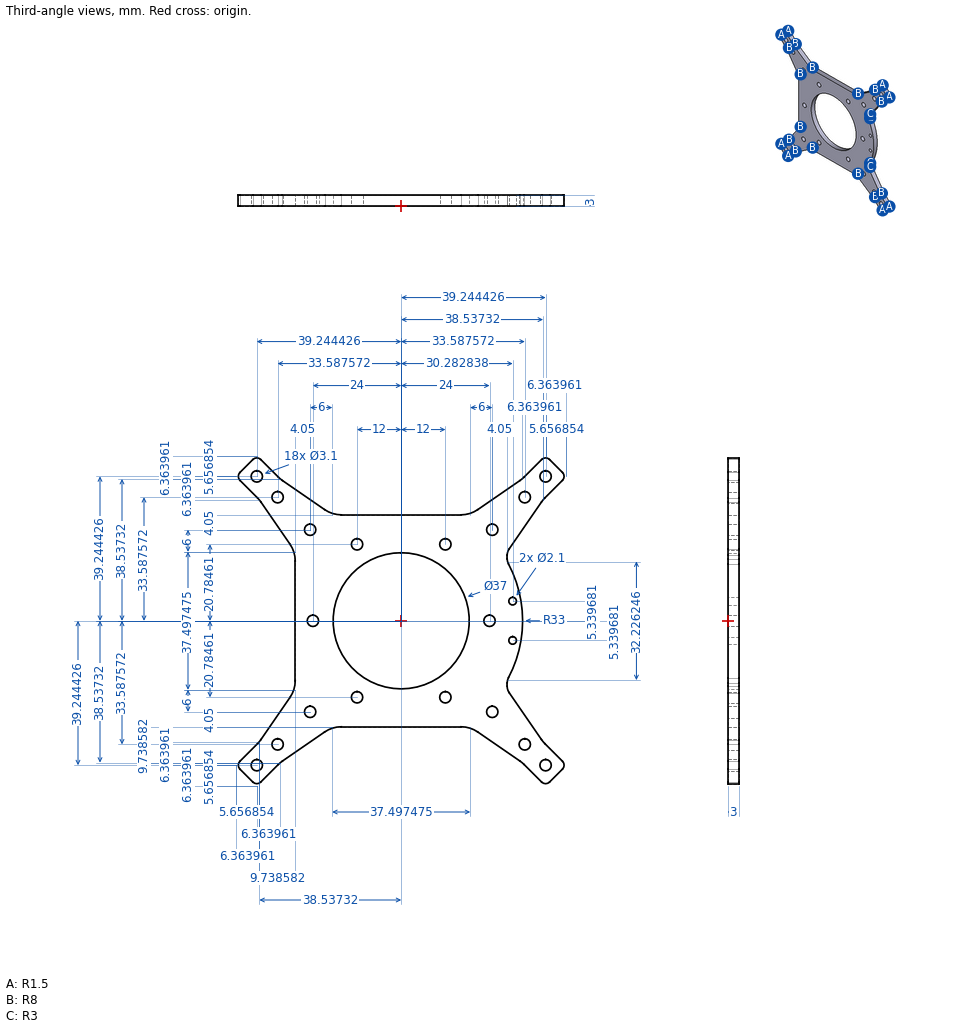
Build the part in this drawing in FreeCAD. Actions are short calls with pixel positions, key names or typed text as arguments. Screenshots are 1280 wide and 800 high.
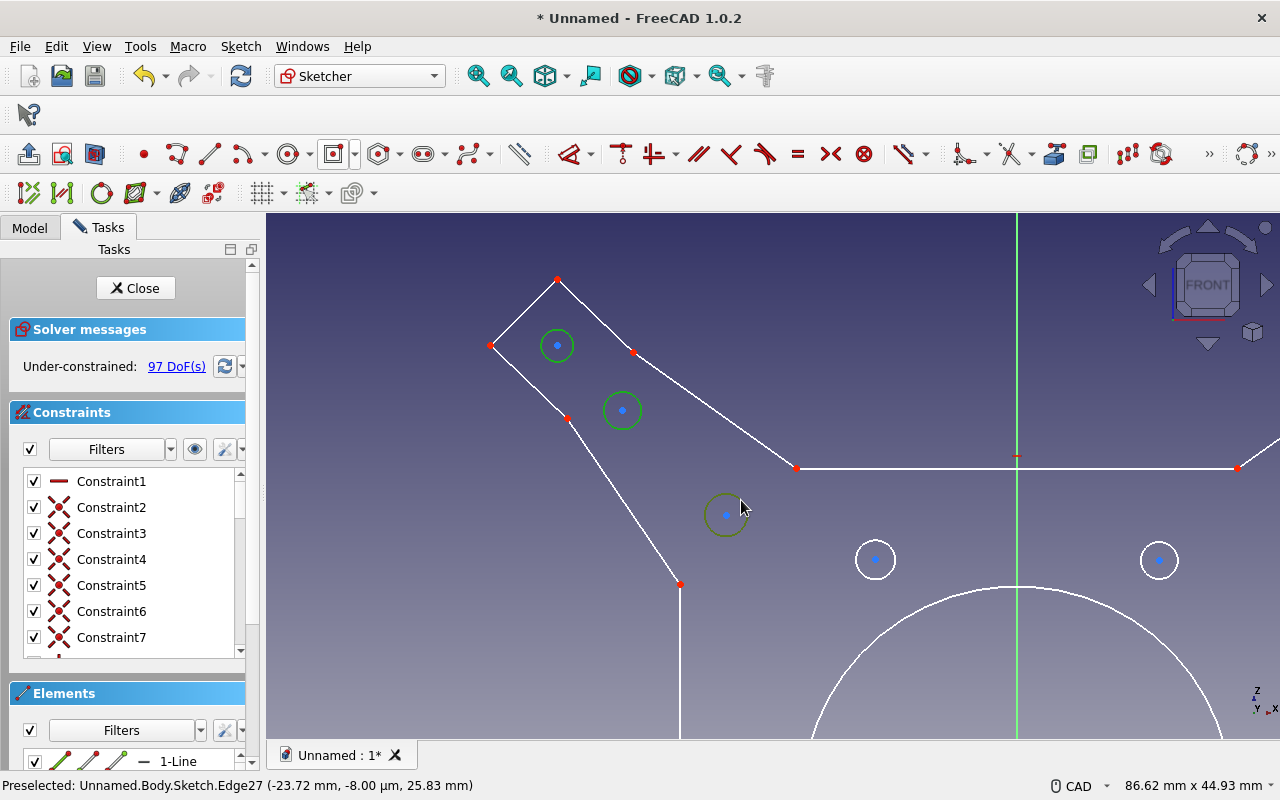
click(889, 546)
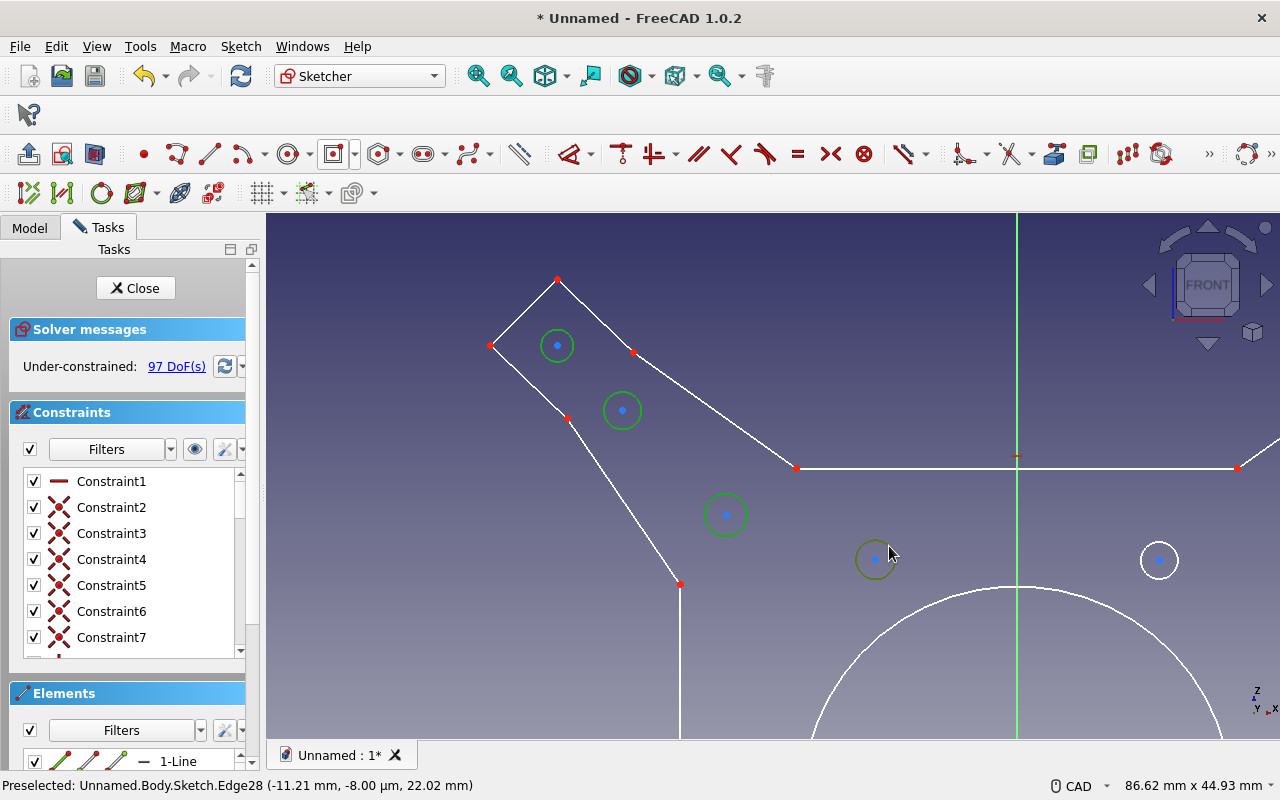
scroll(570, 336, down, 6)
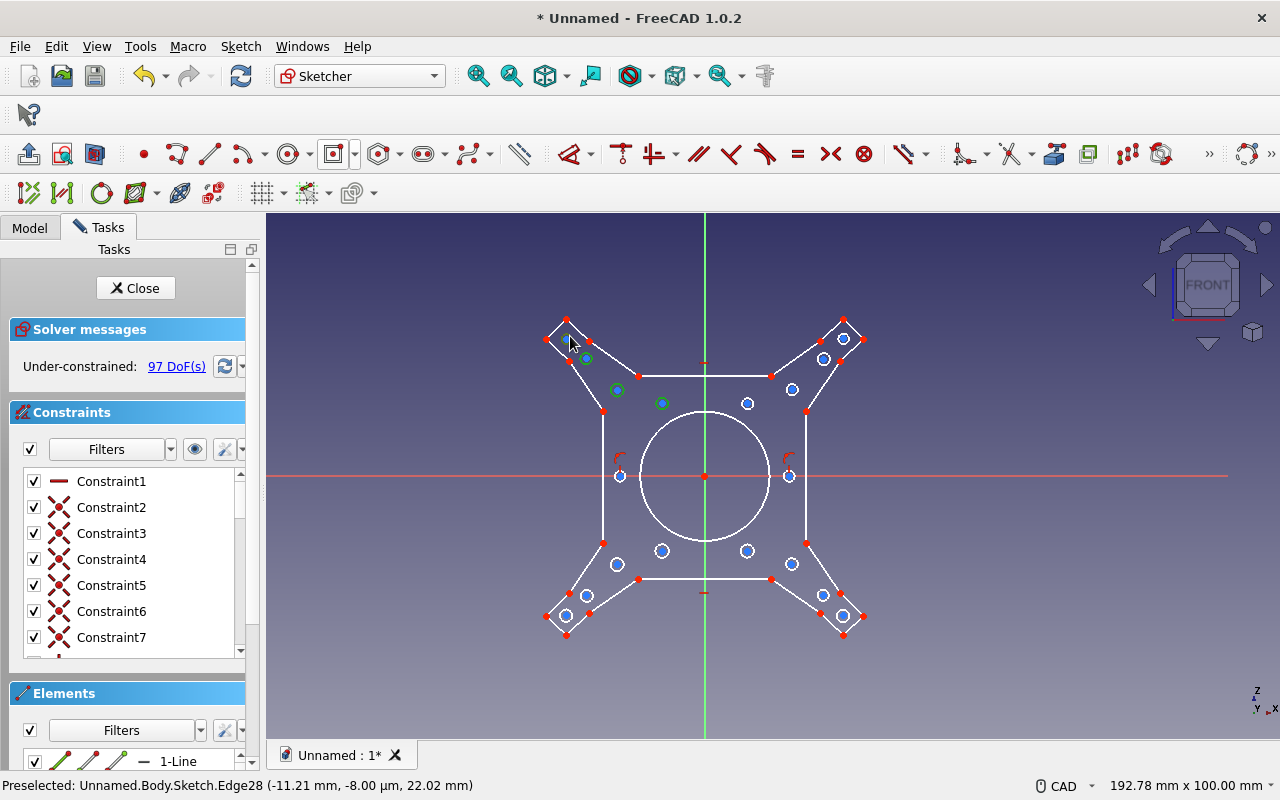
scroll(752, 400, up, 5)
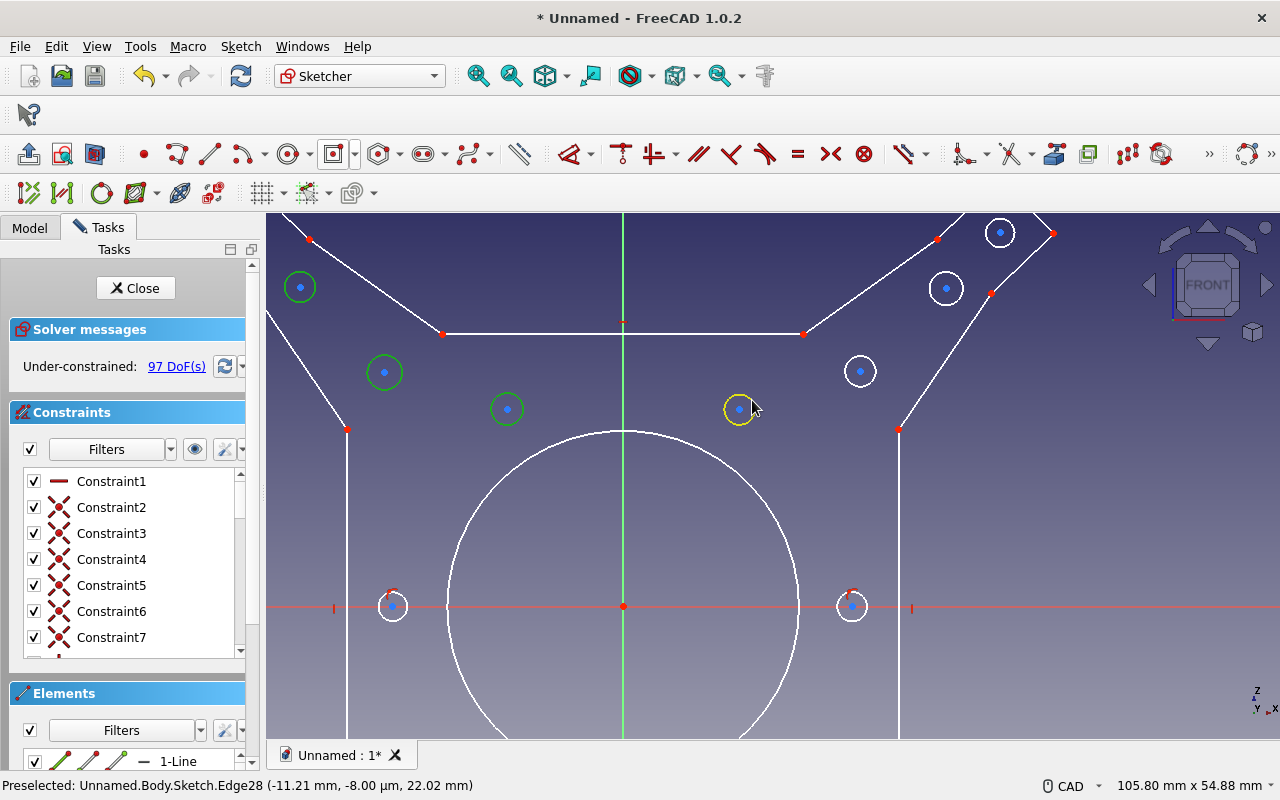
click(750, 399)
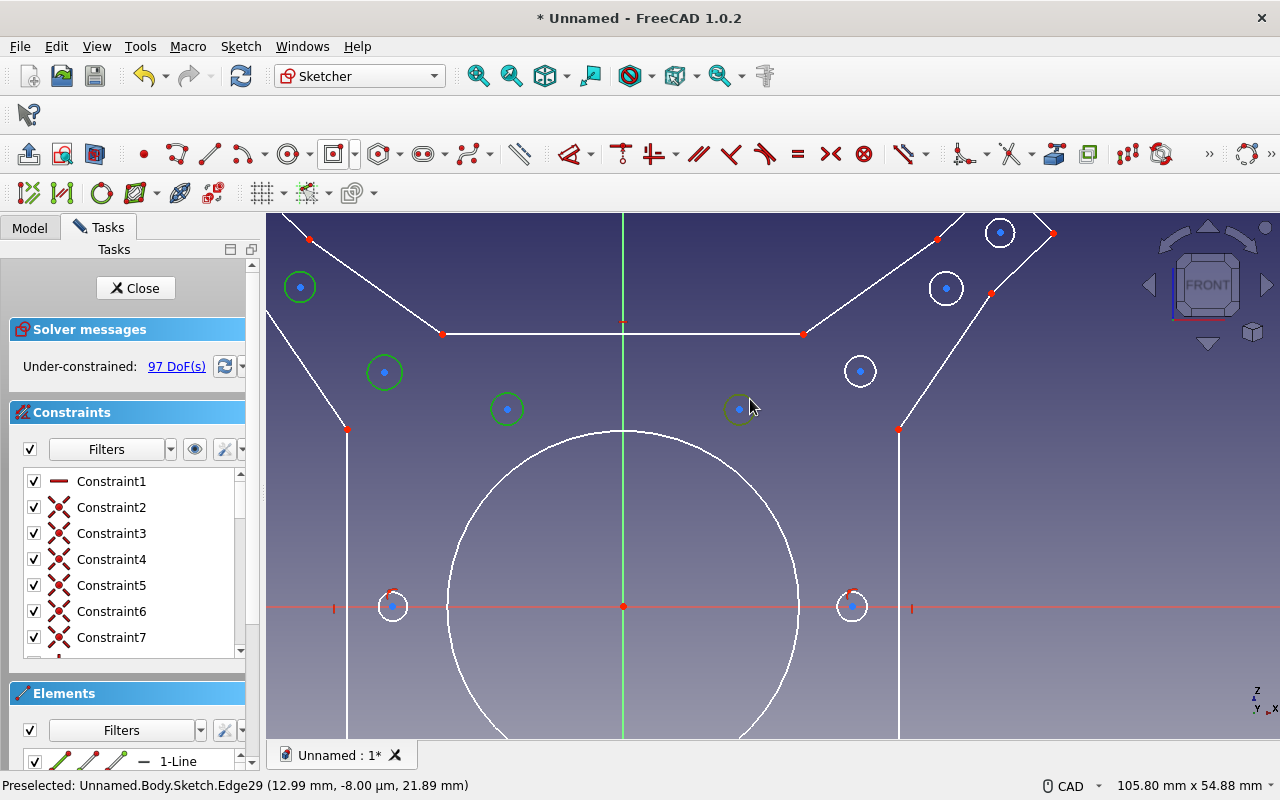
click(990, 243)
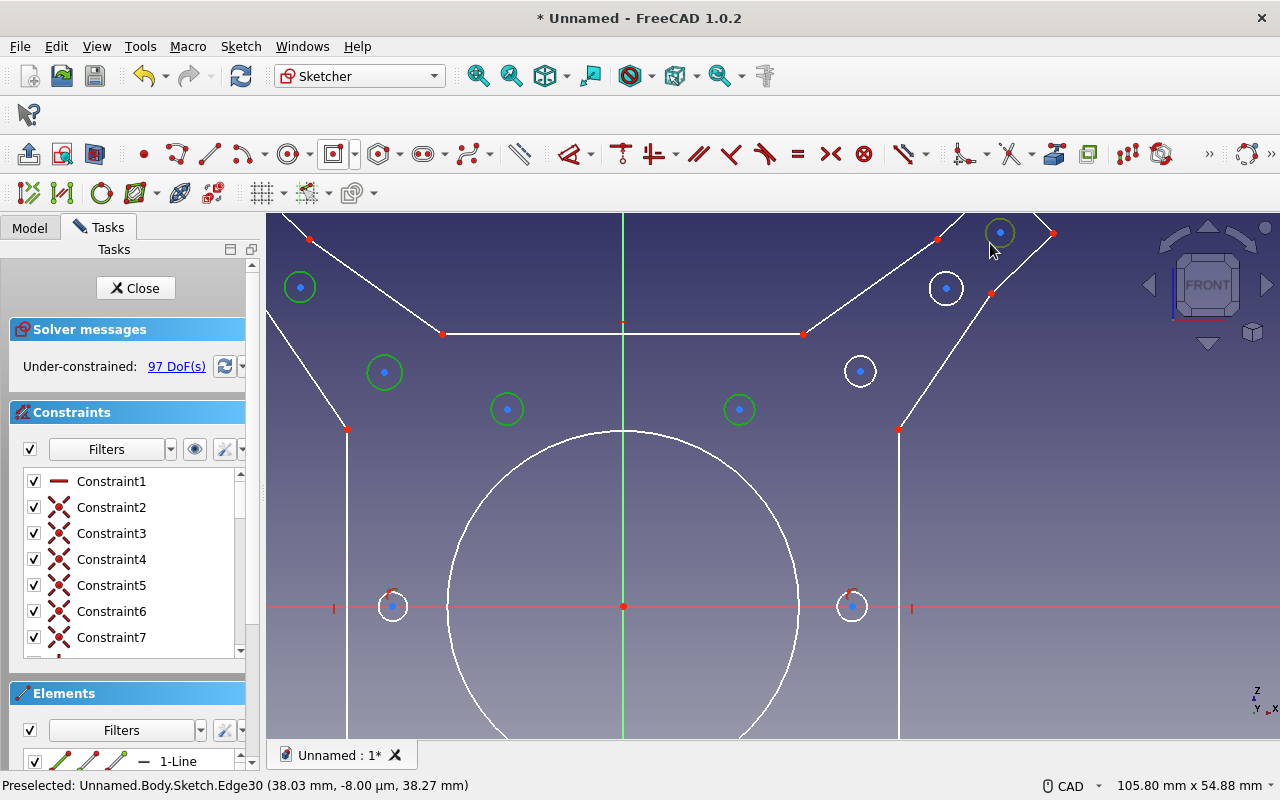
click(958, 277)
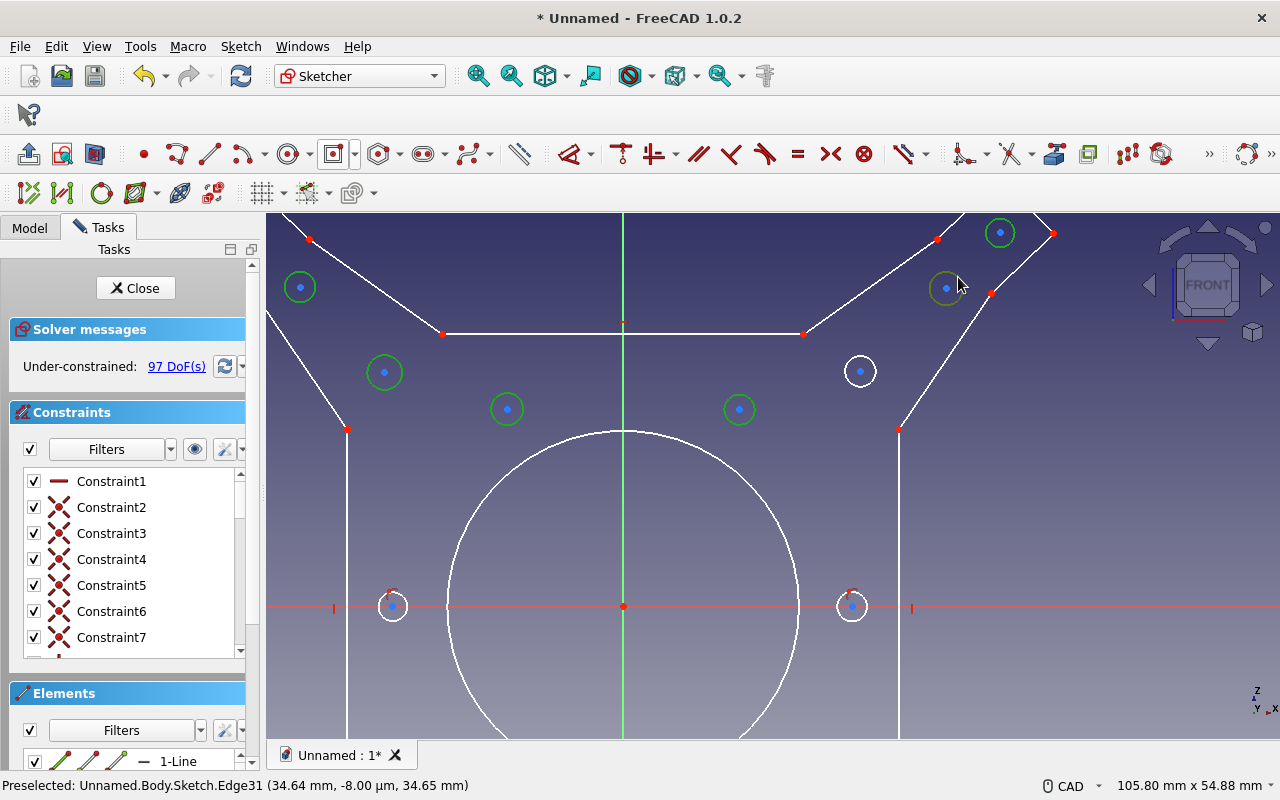
click(871, 361)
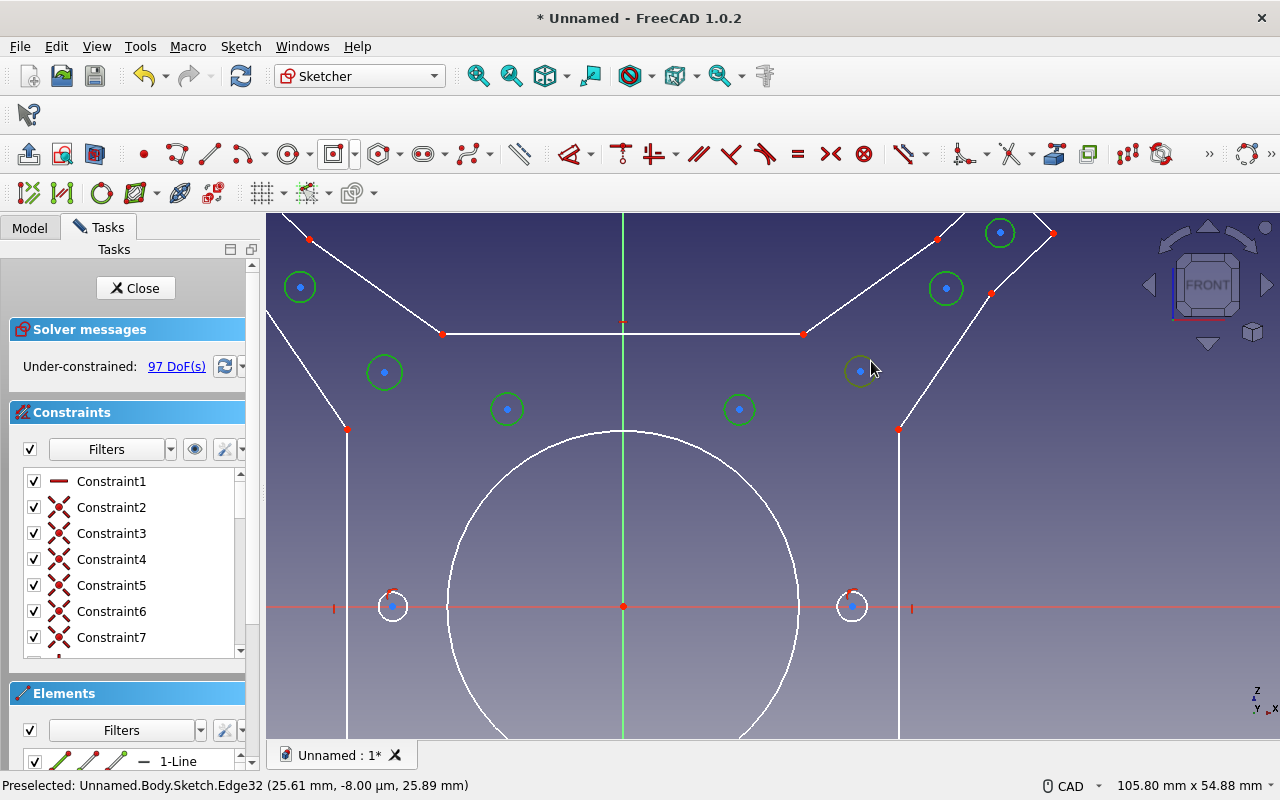
scroll(403, 597, up, 2)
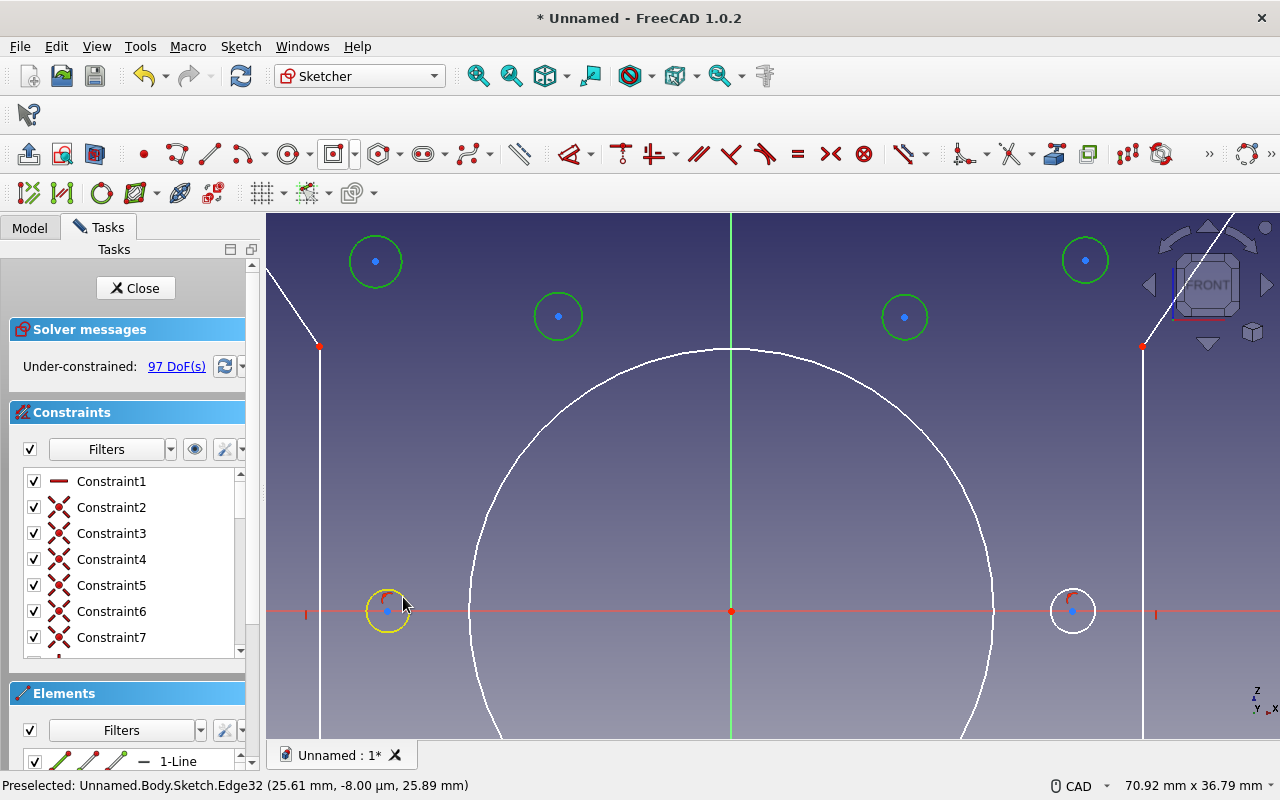
click(403, 596)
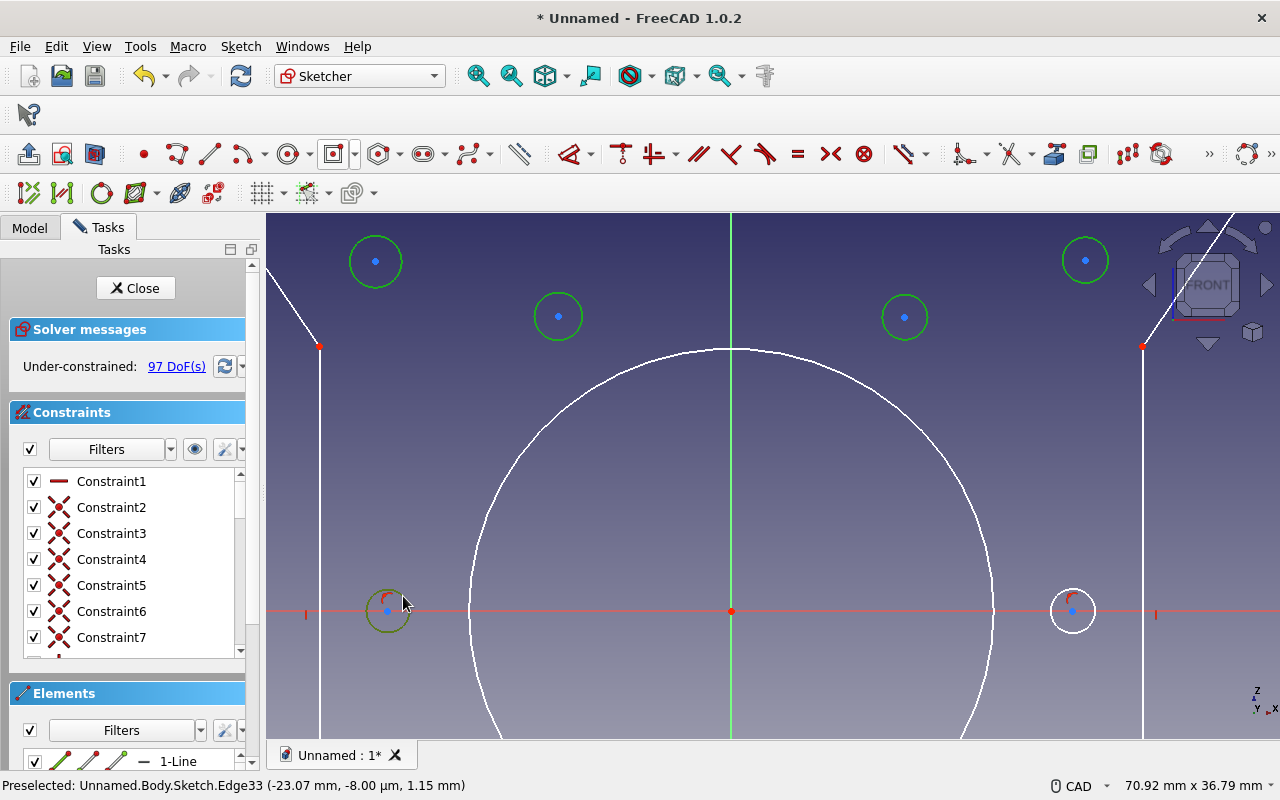
scroll(696, 432, down, 7)